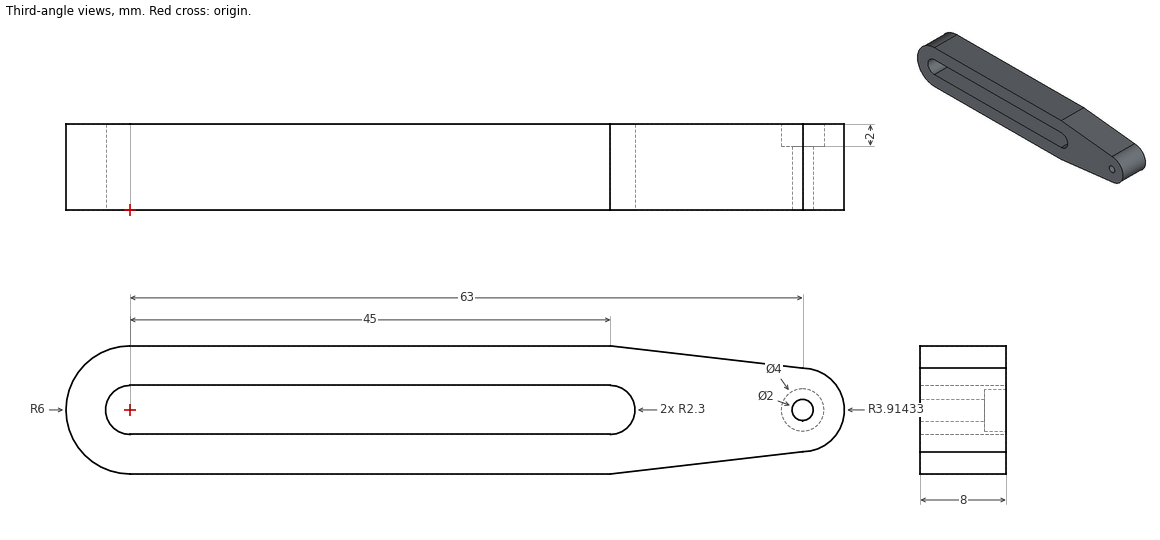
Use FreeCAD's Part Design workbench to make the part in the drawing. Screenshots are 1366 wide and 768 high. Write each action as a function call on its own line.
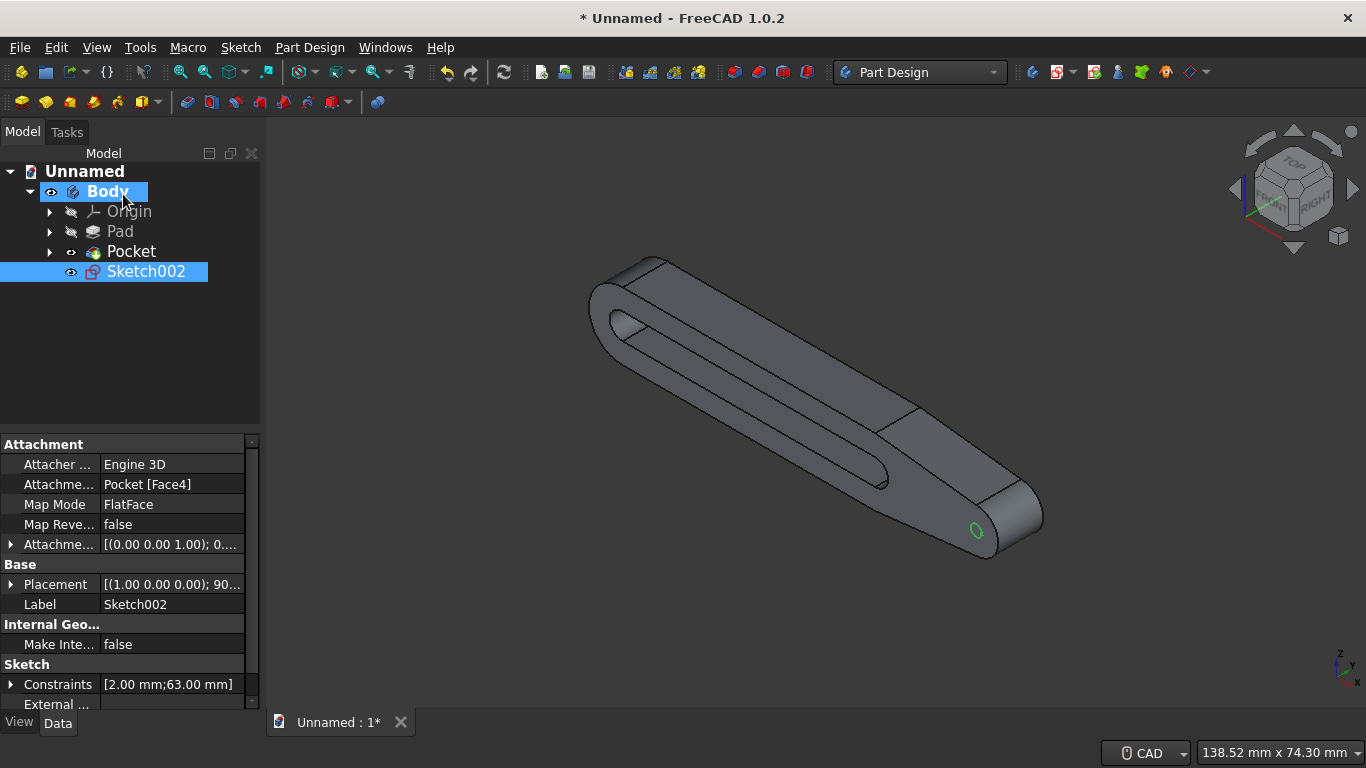
click(188, 102)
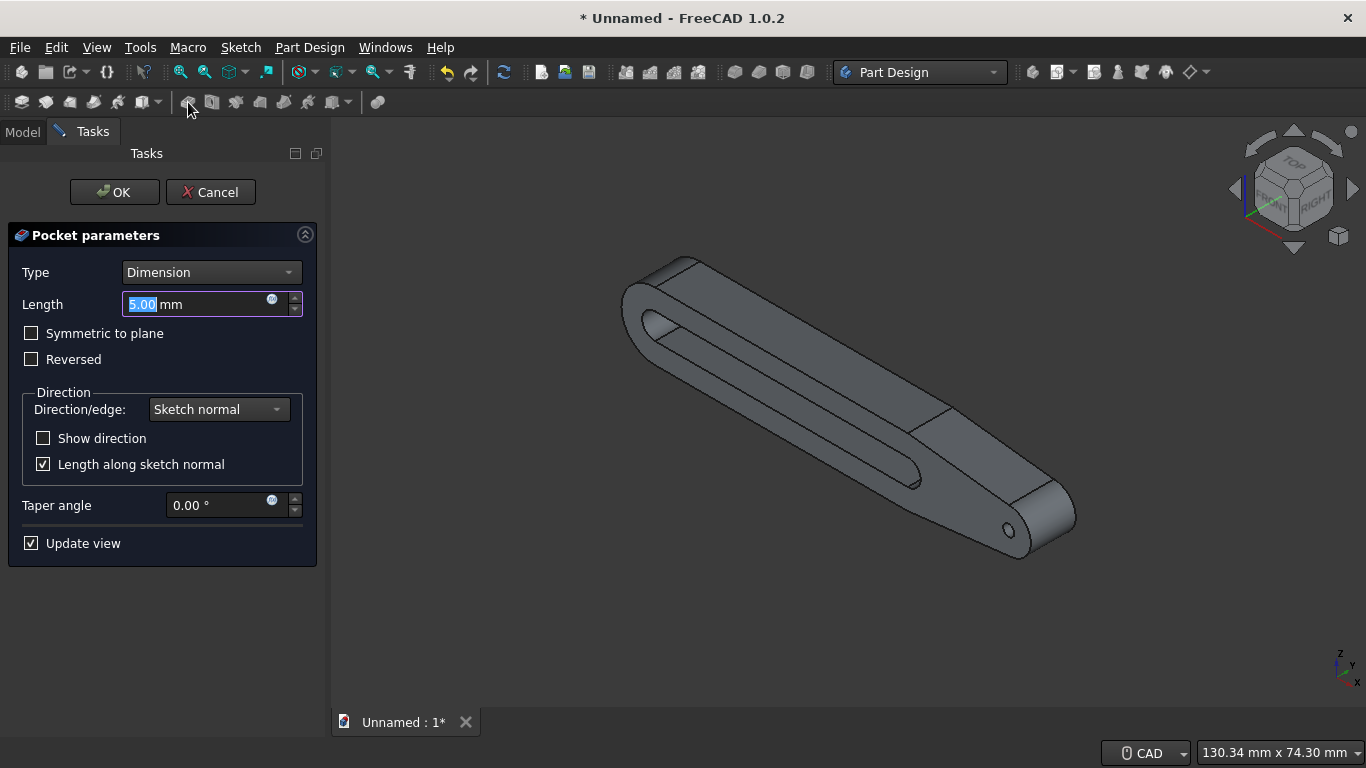
click(212, 272)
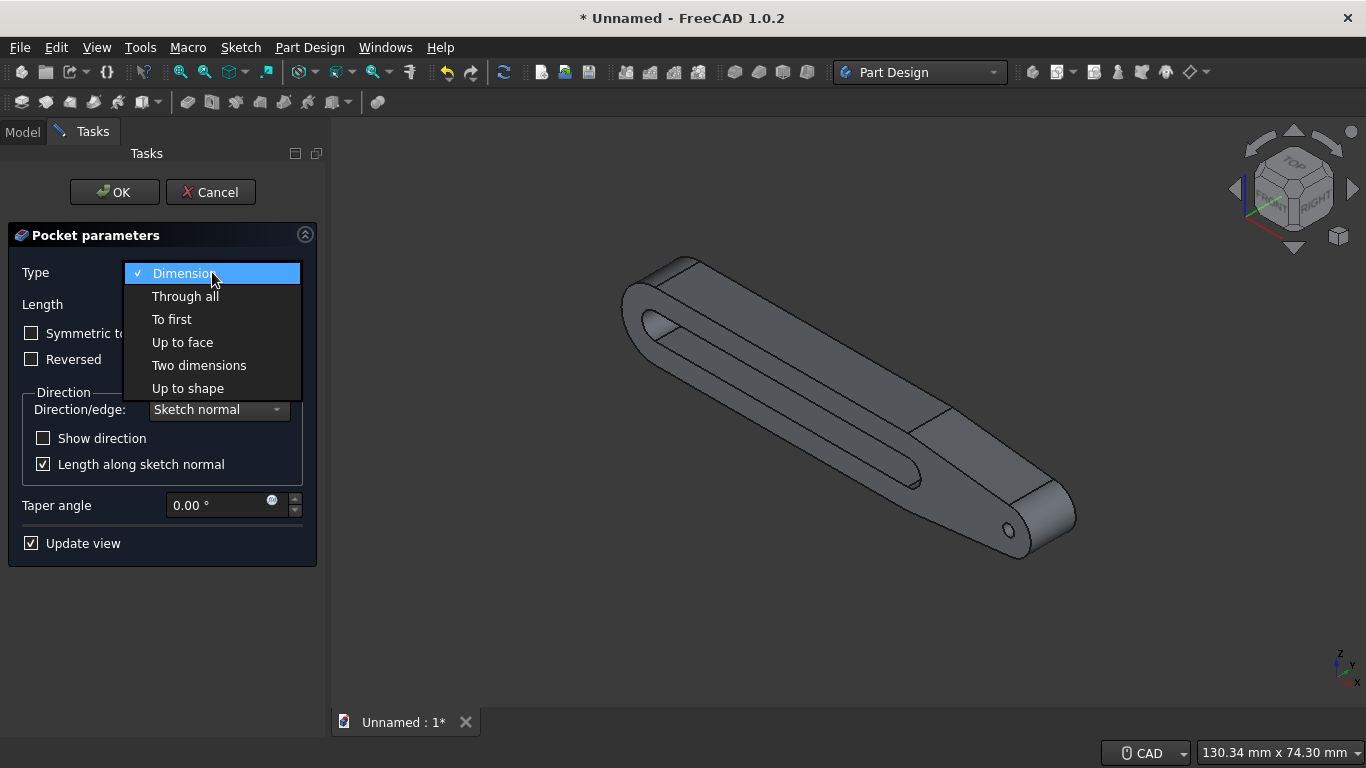
click(212, 296)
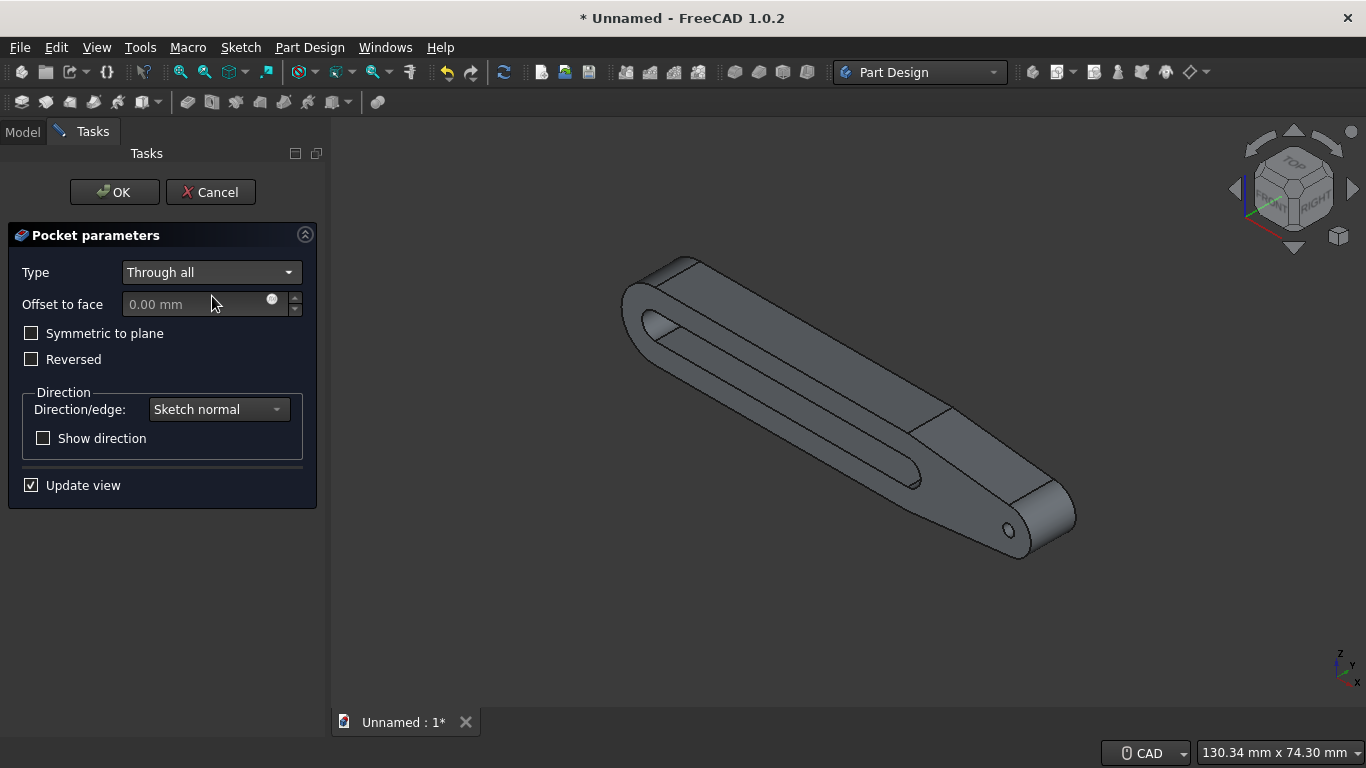
click(115, 192)